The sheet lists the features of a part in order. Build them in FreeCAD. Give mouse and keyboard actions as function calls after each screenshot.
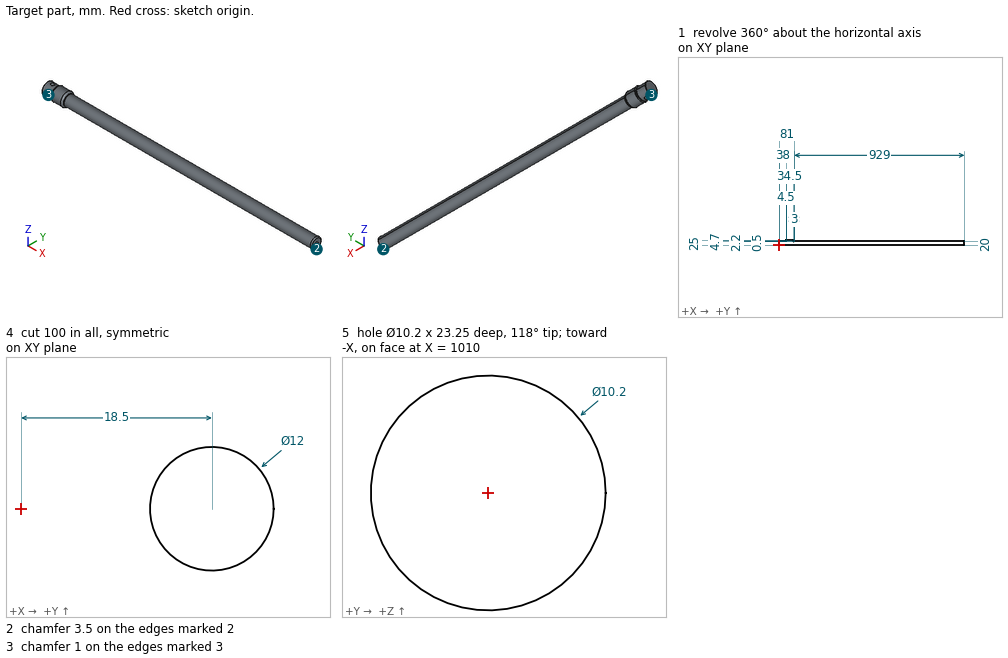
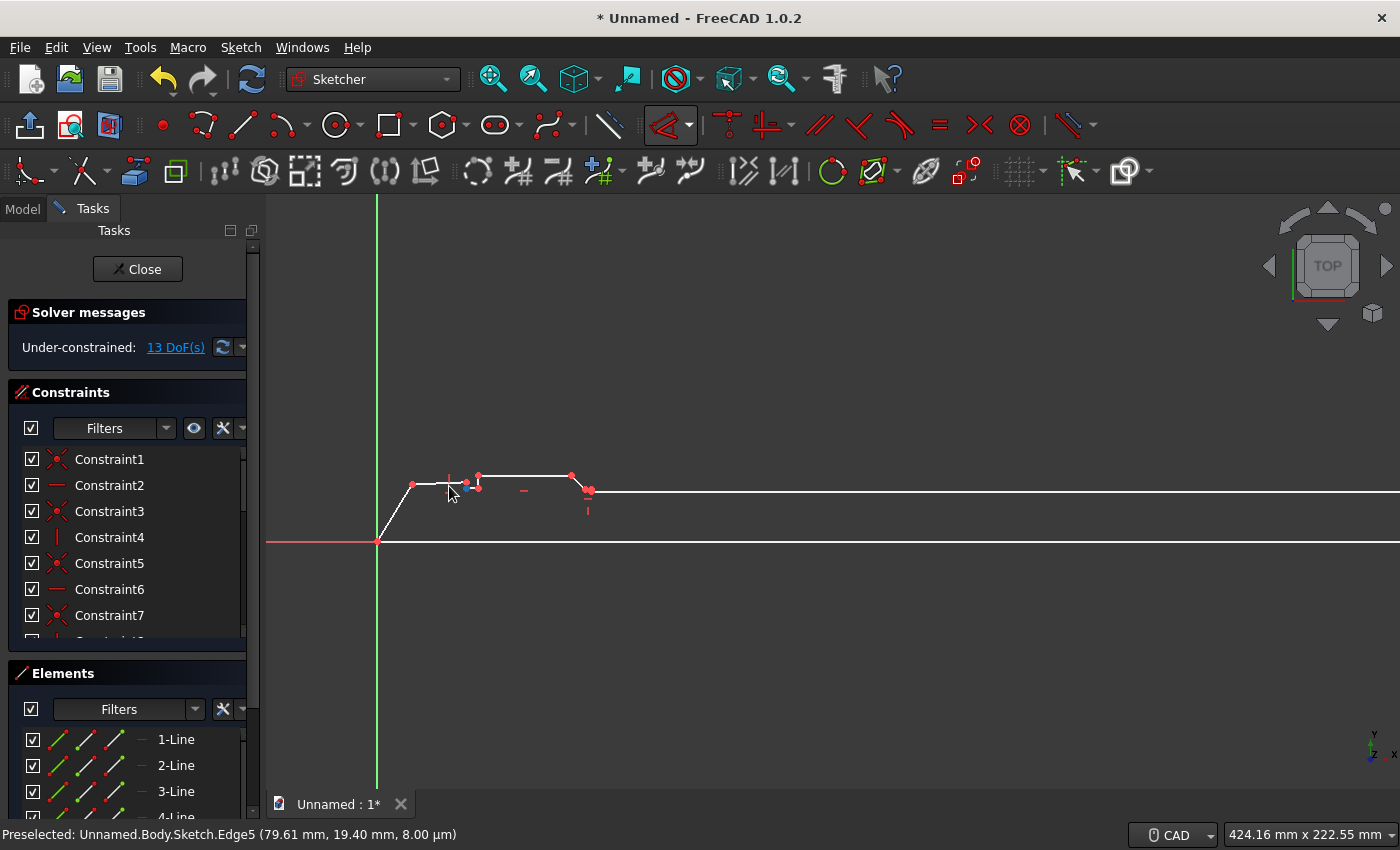
click(428, 484)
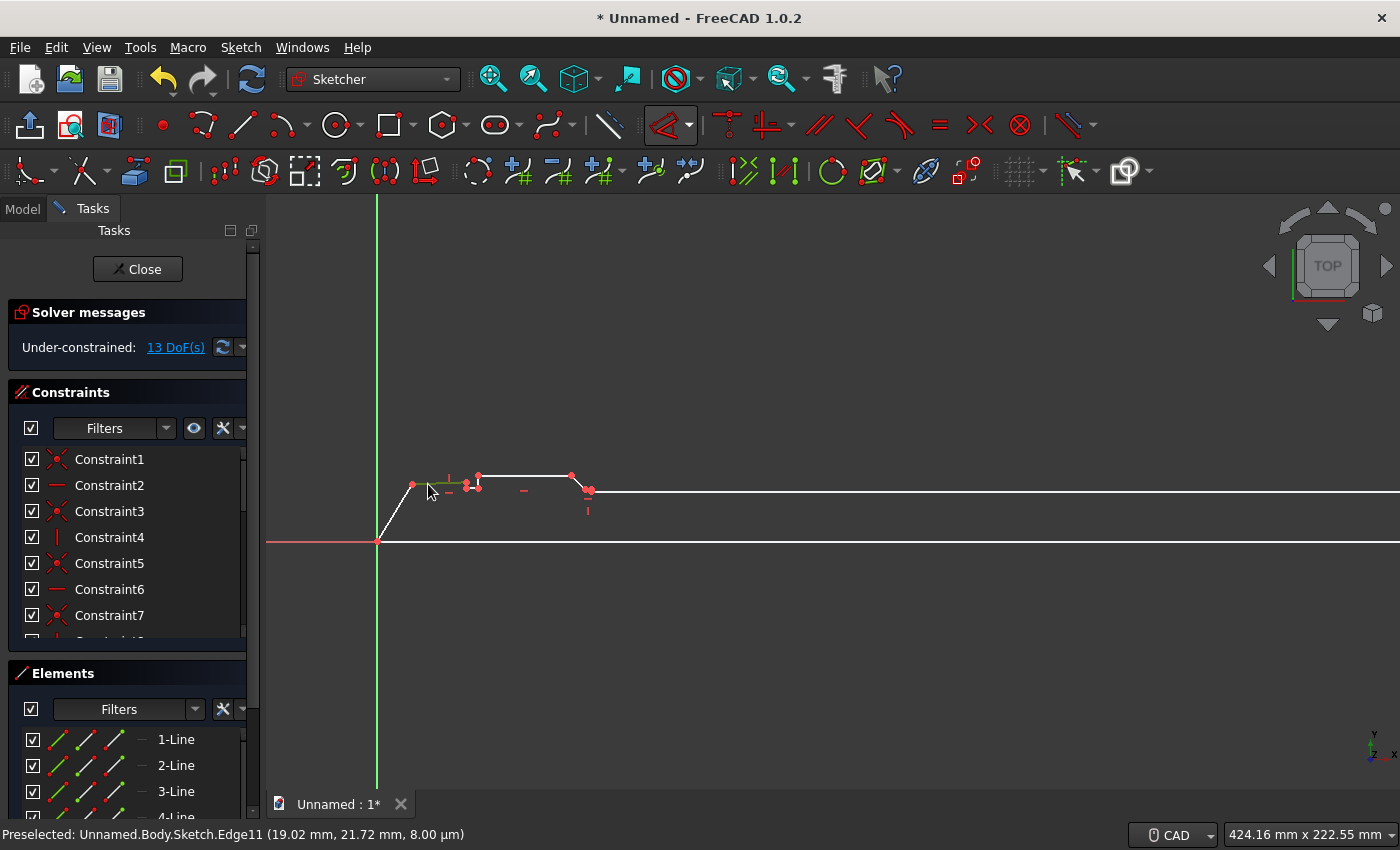
click(794, 126)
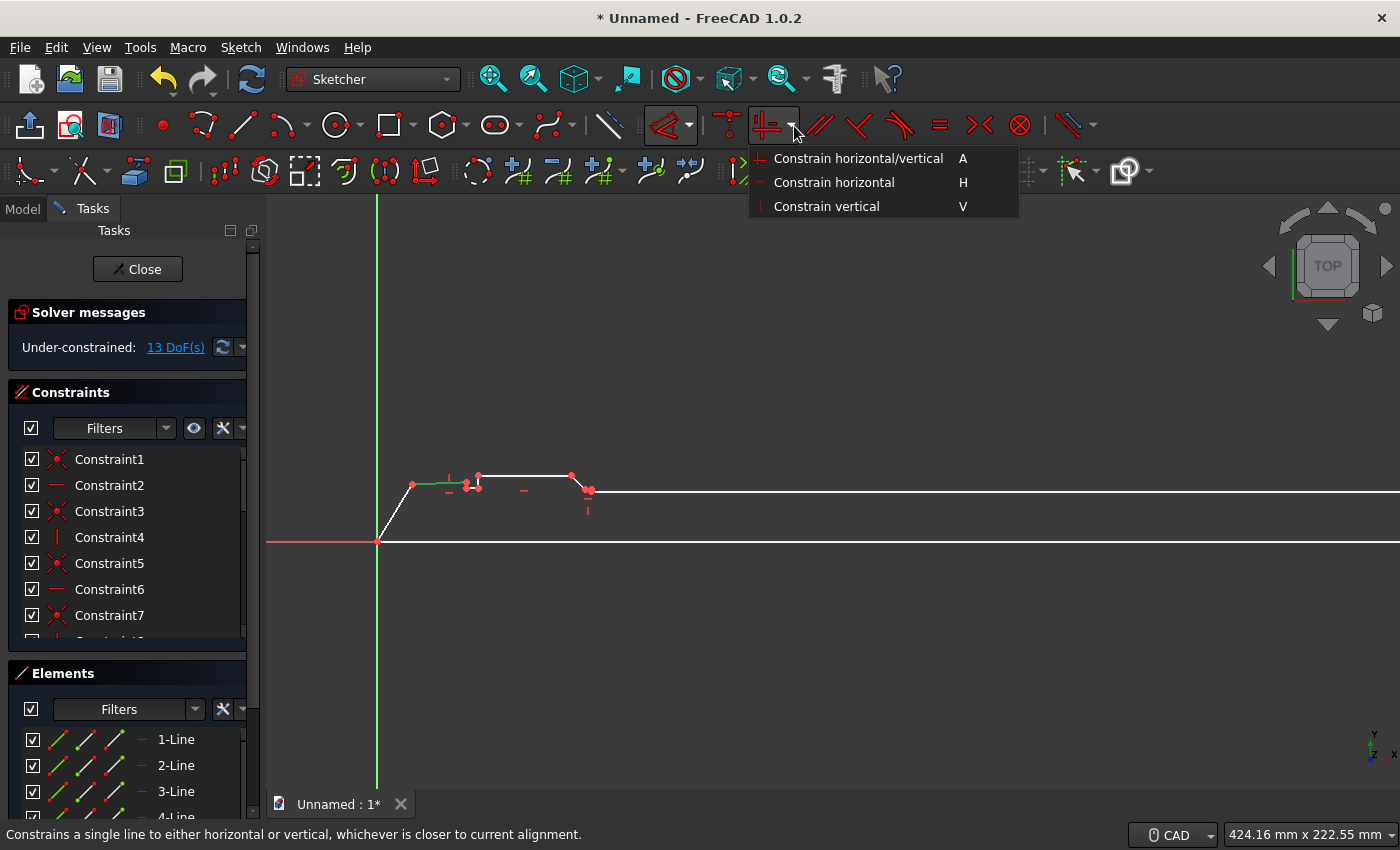
click(884, 182)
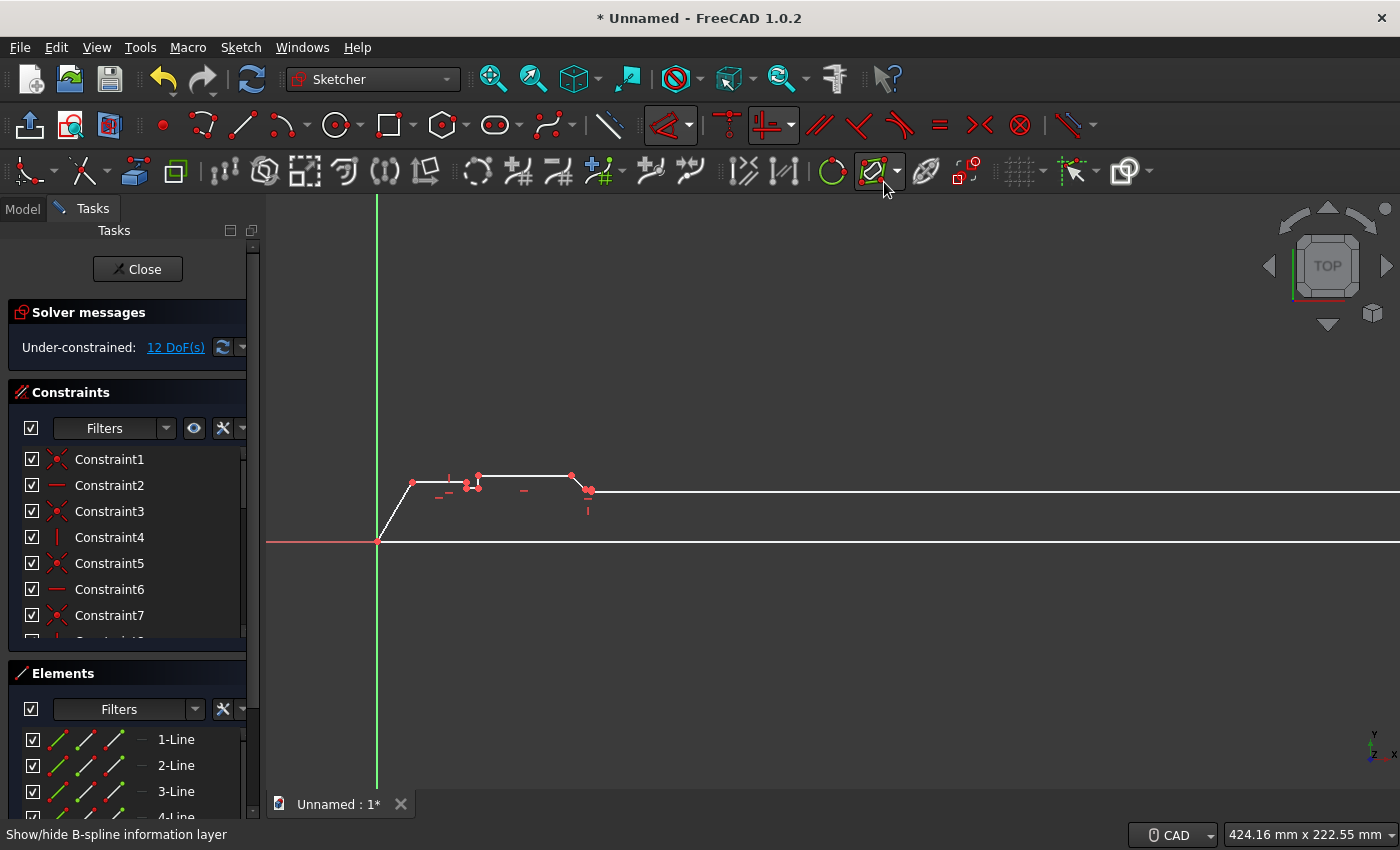
click(402, 500)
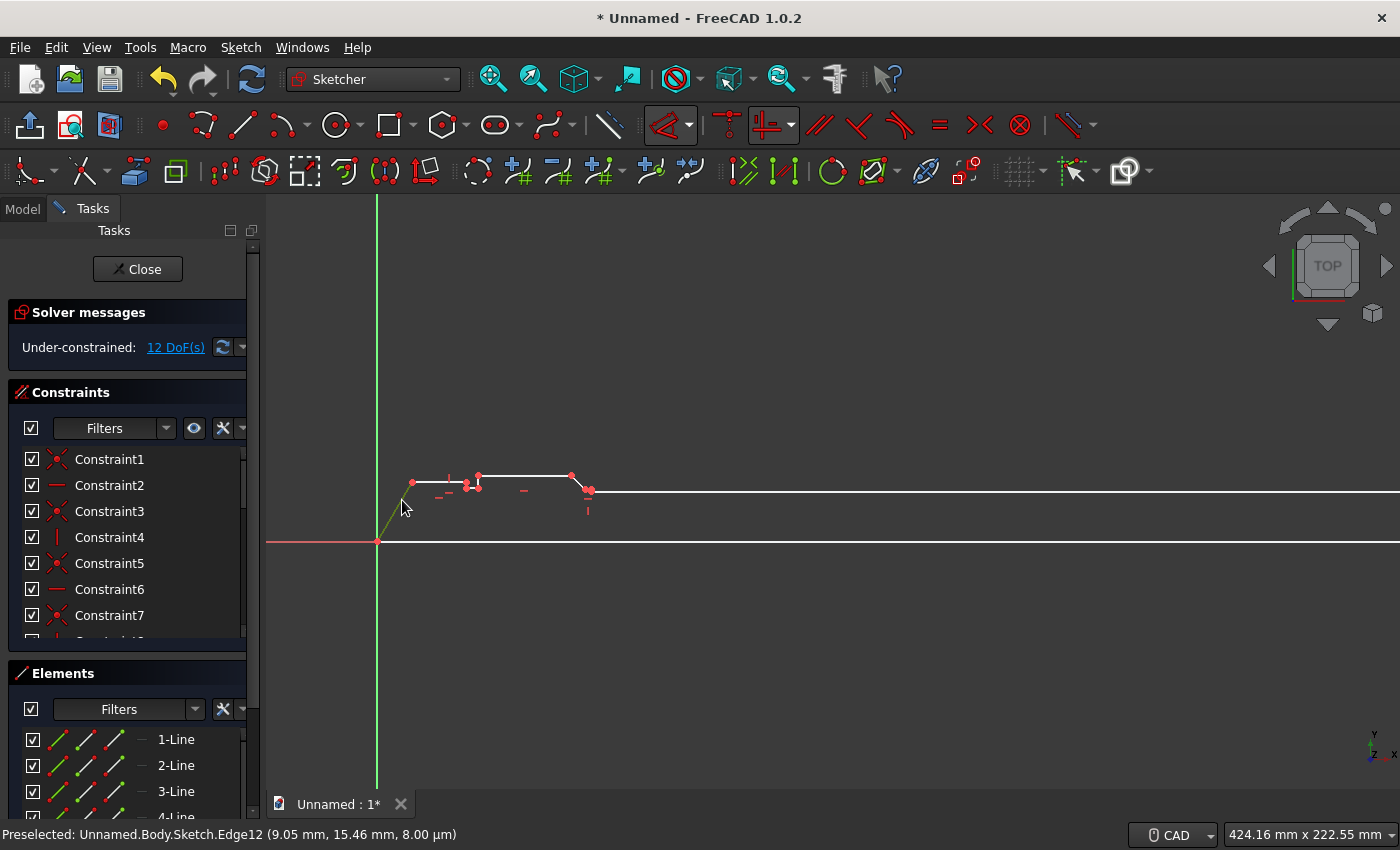
click(794, 126)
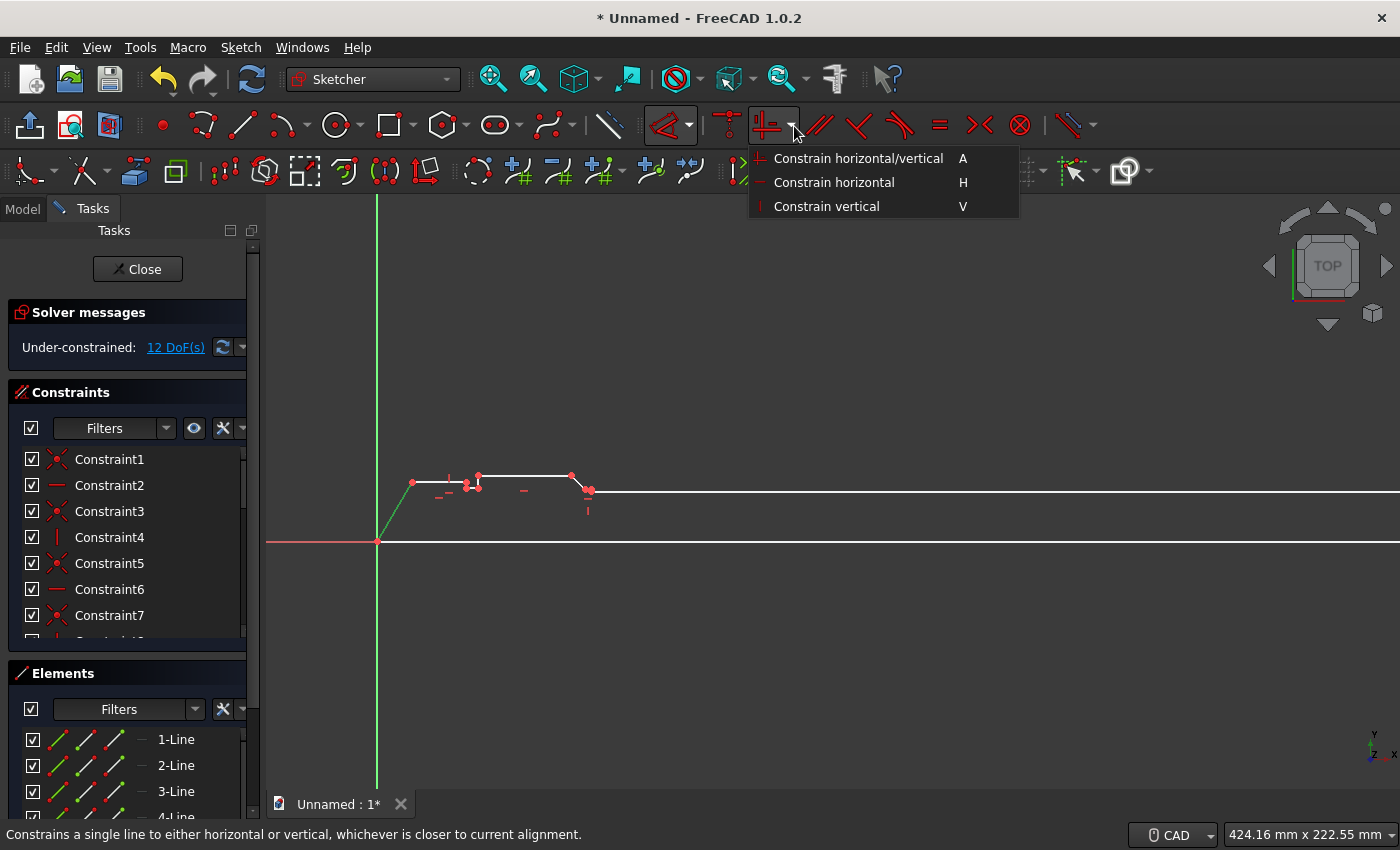
click(884, 206)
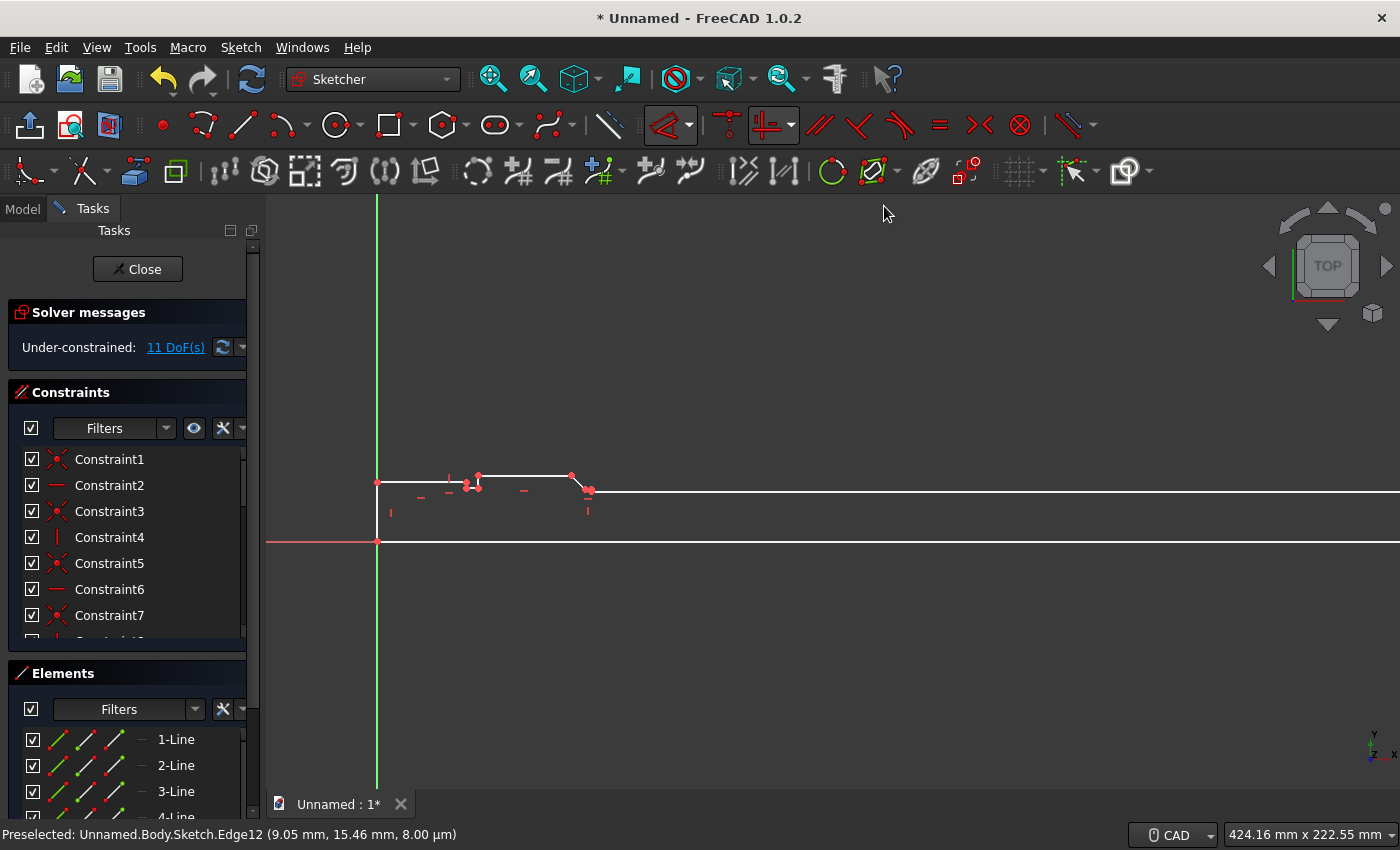
click(664, 126)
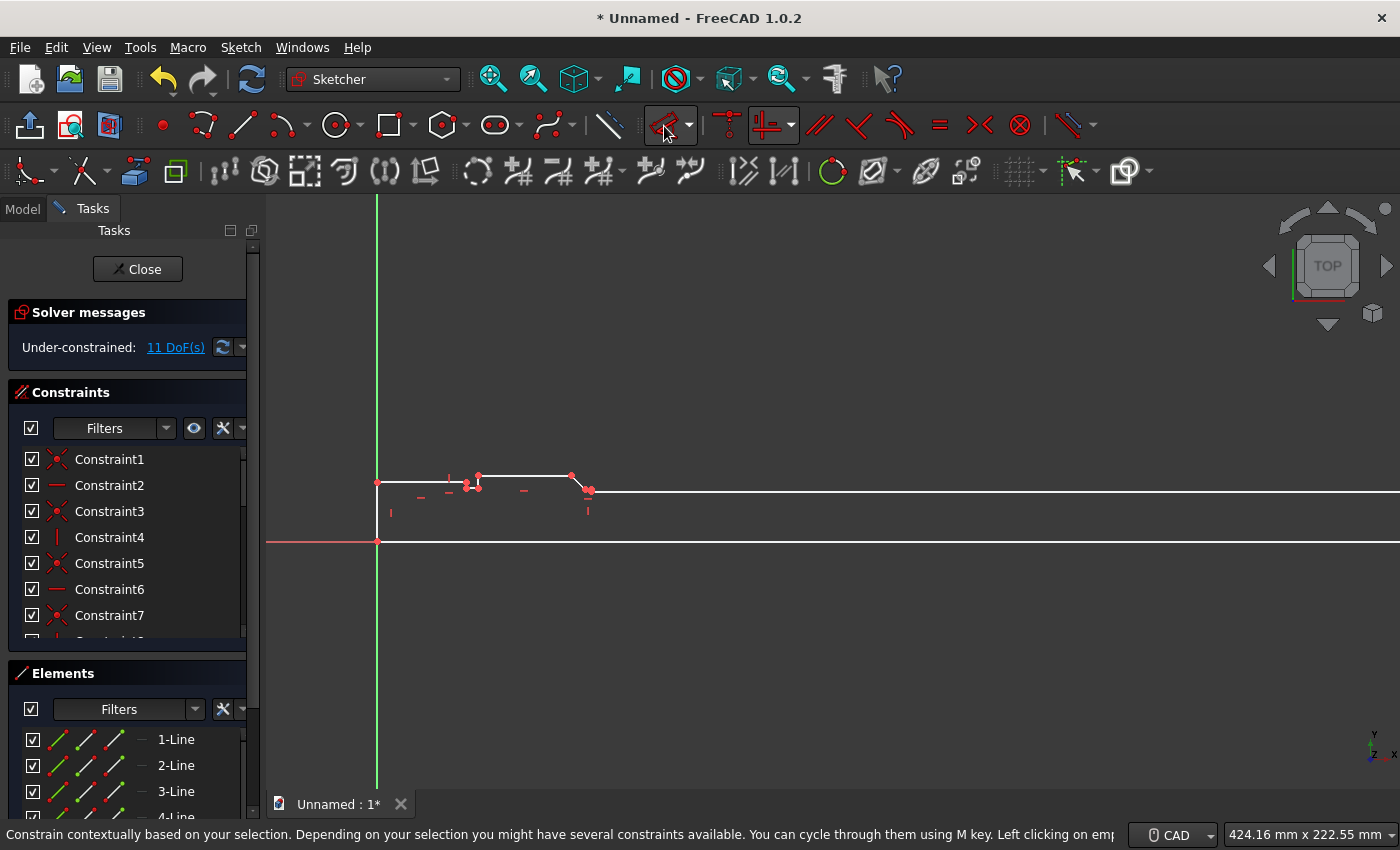
scroll(589, 490, up, 8)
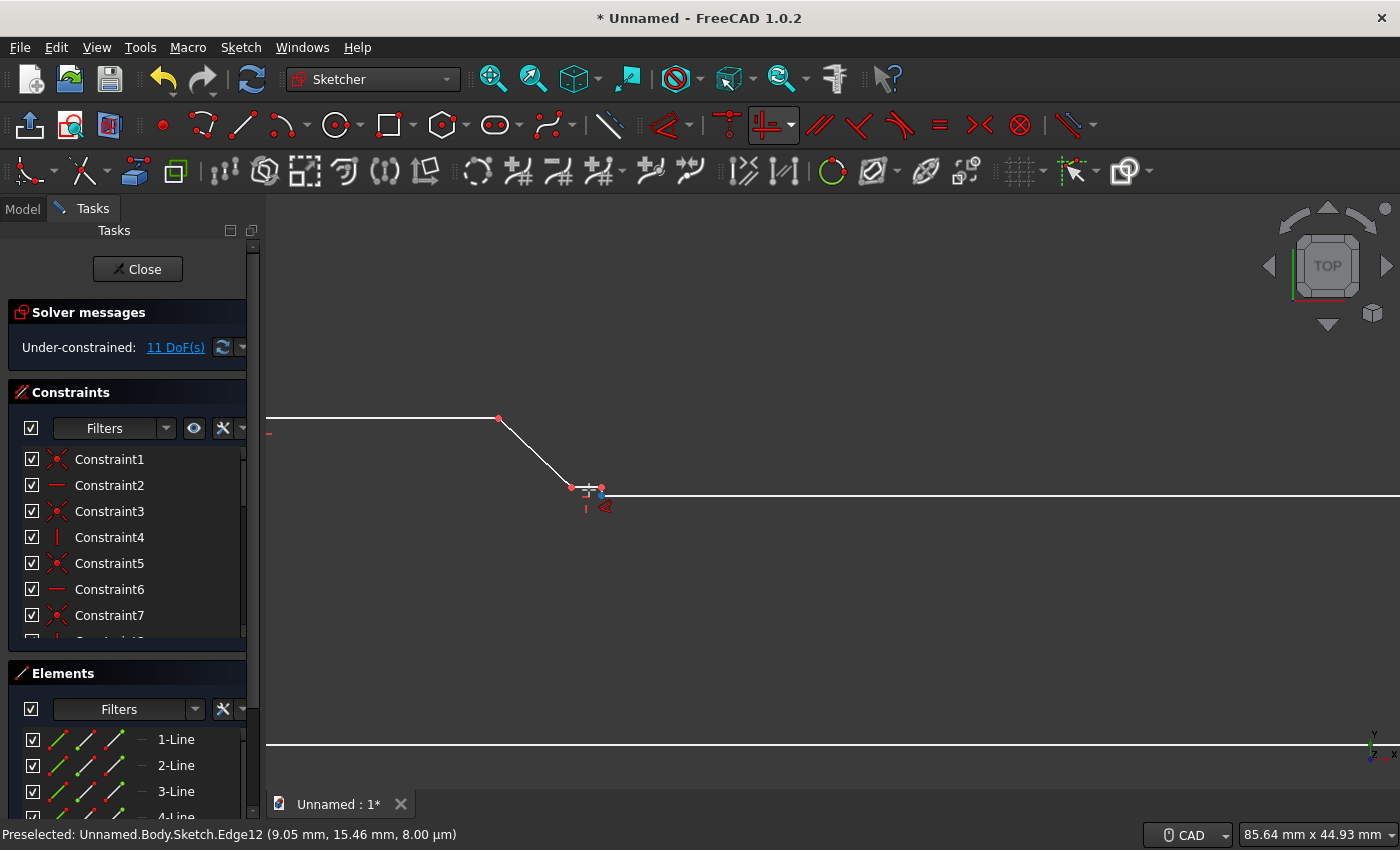
click(587, 487)
click(587, 453)